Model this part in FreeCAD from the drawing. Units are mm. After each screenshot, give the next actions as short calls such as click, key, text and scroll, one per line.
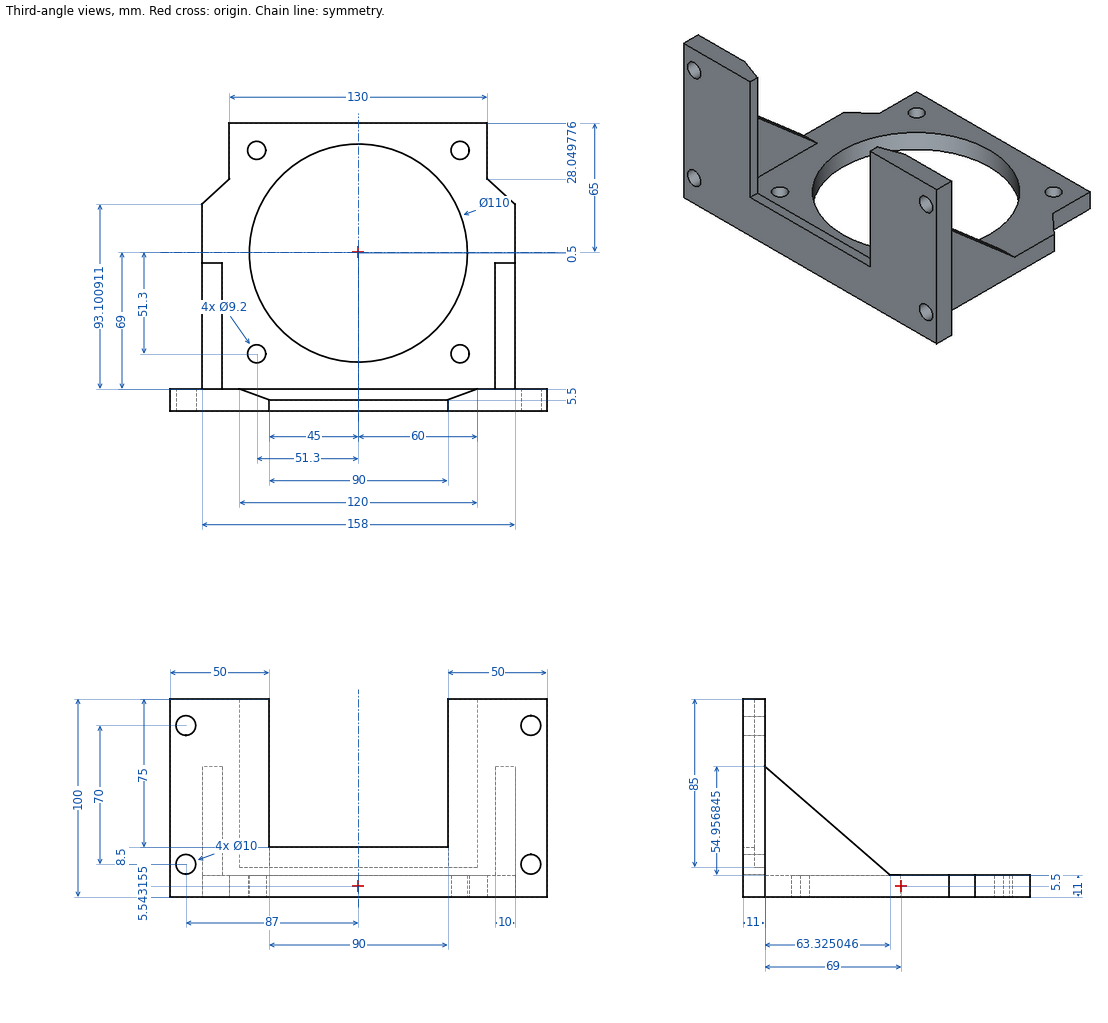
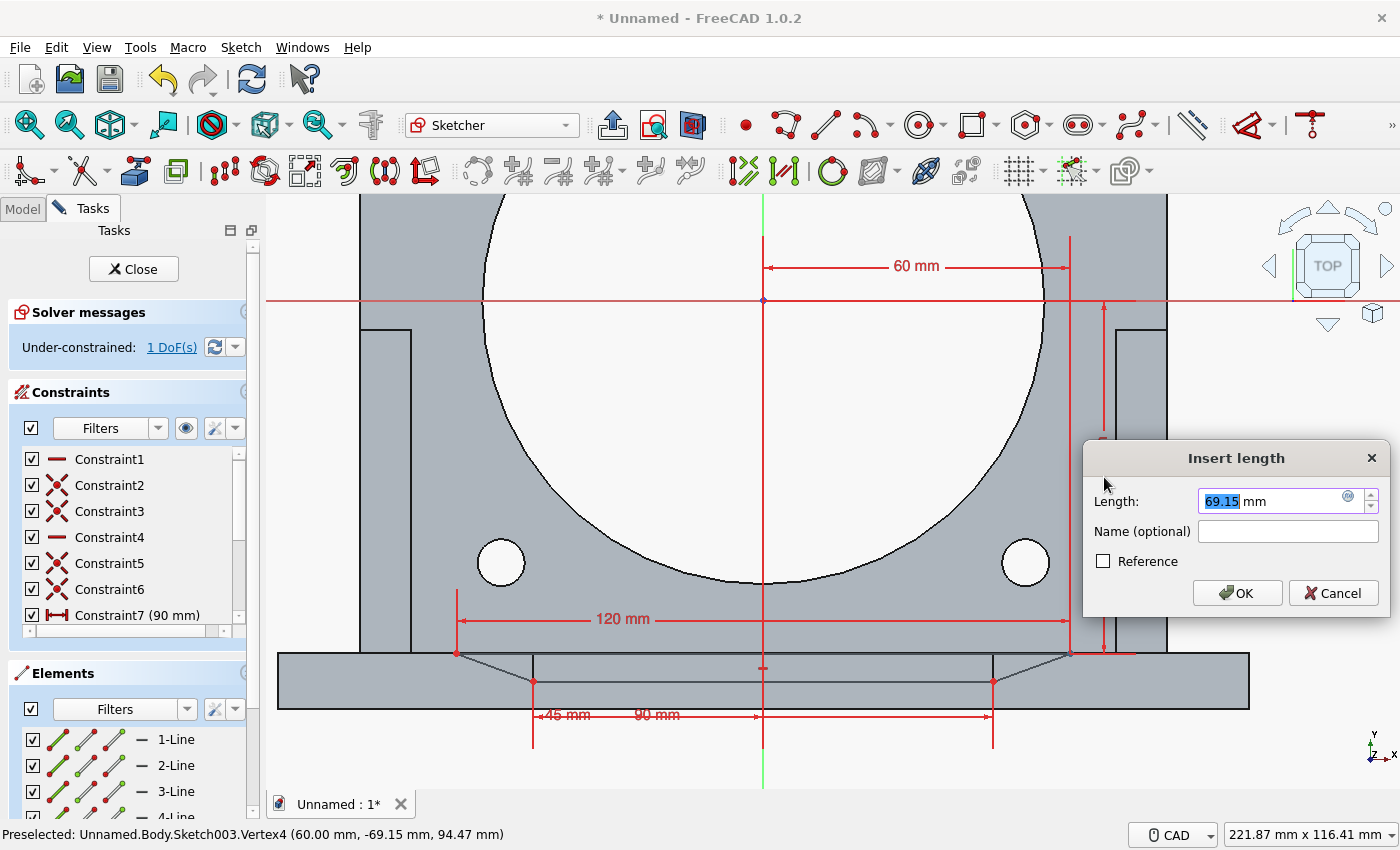
text(69)
key(Return)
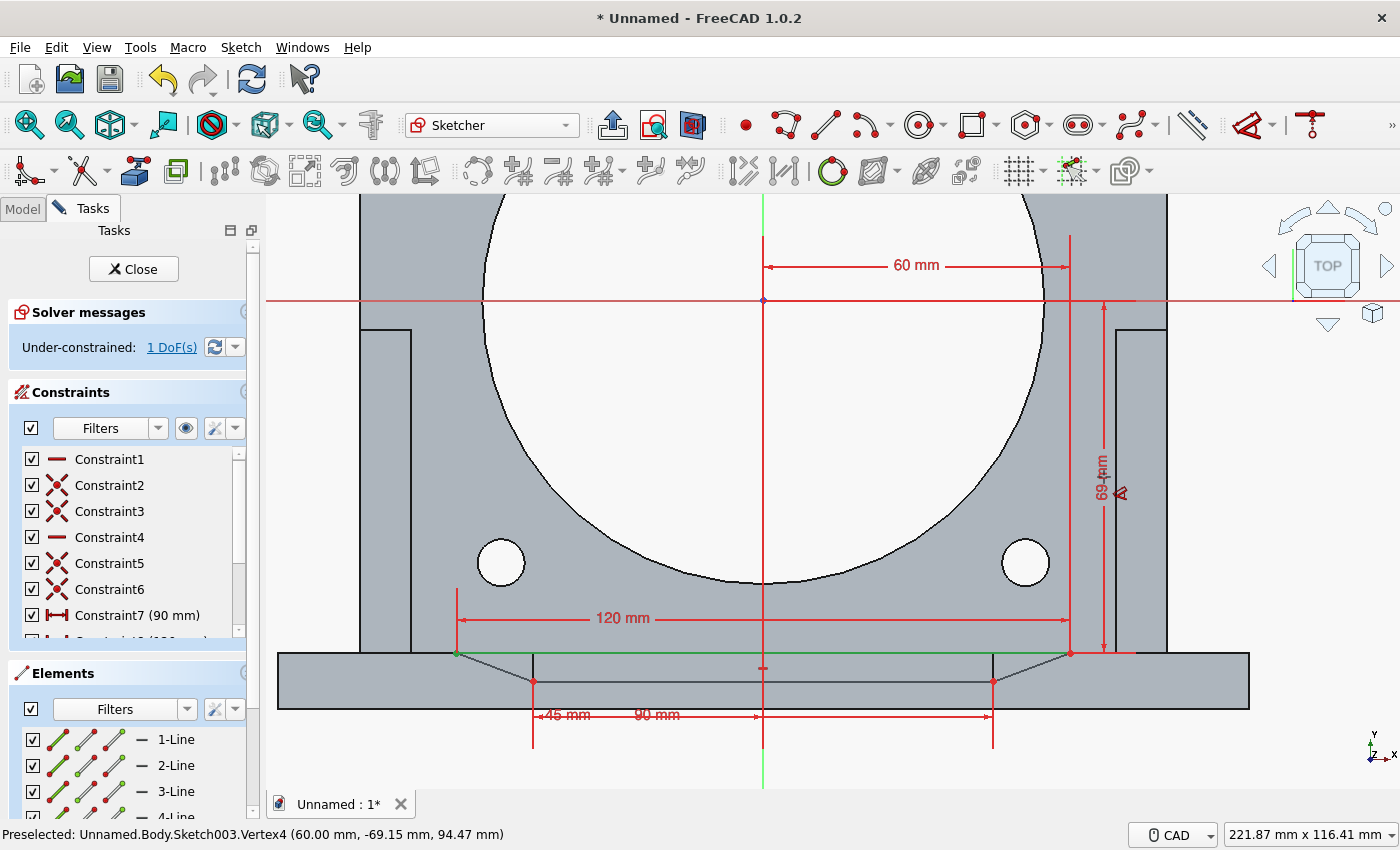
scroll(1016, 673, up, 2)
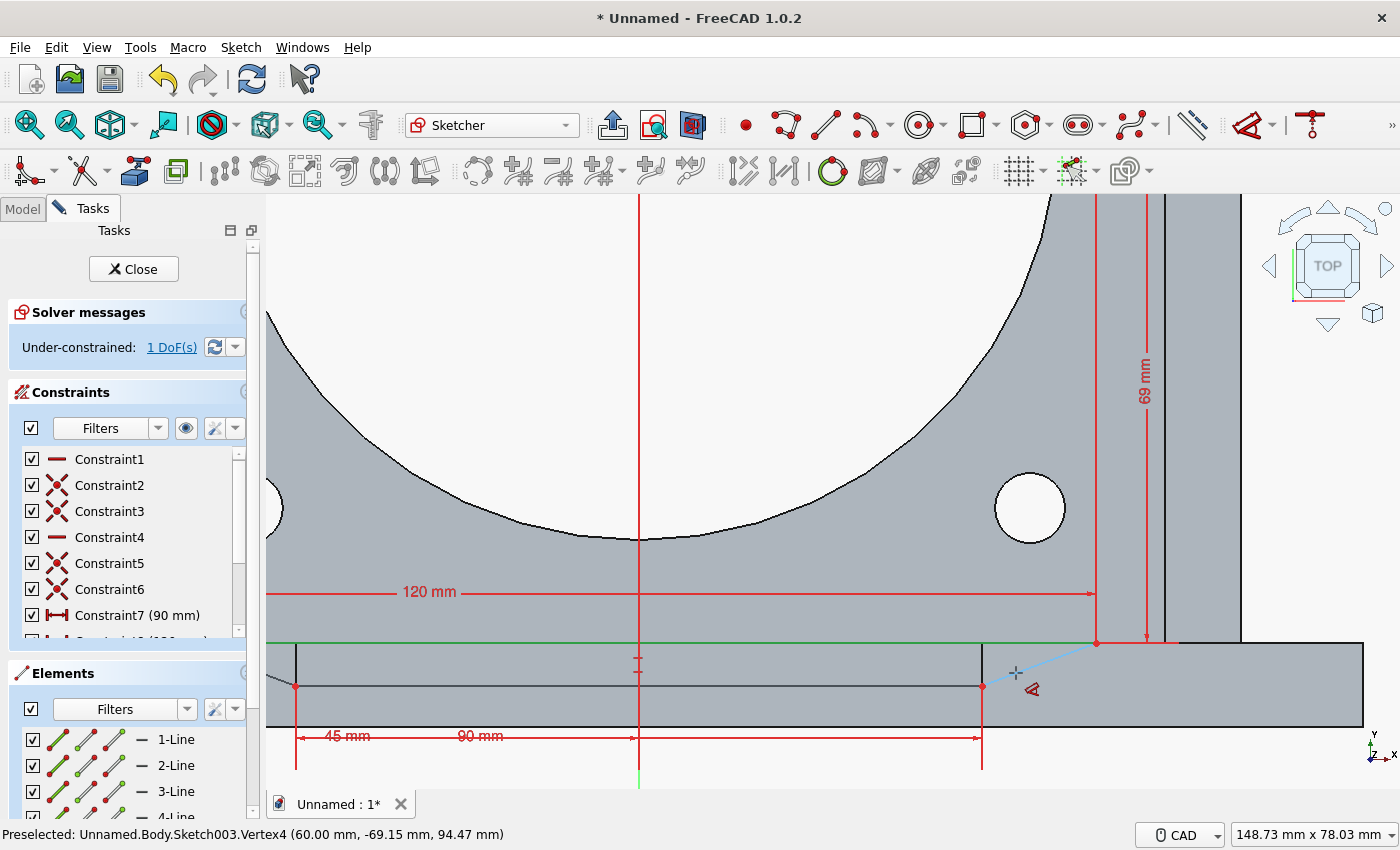
click(1016, 673)
click(1130, 665)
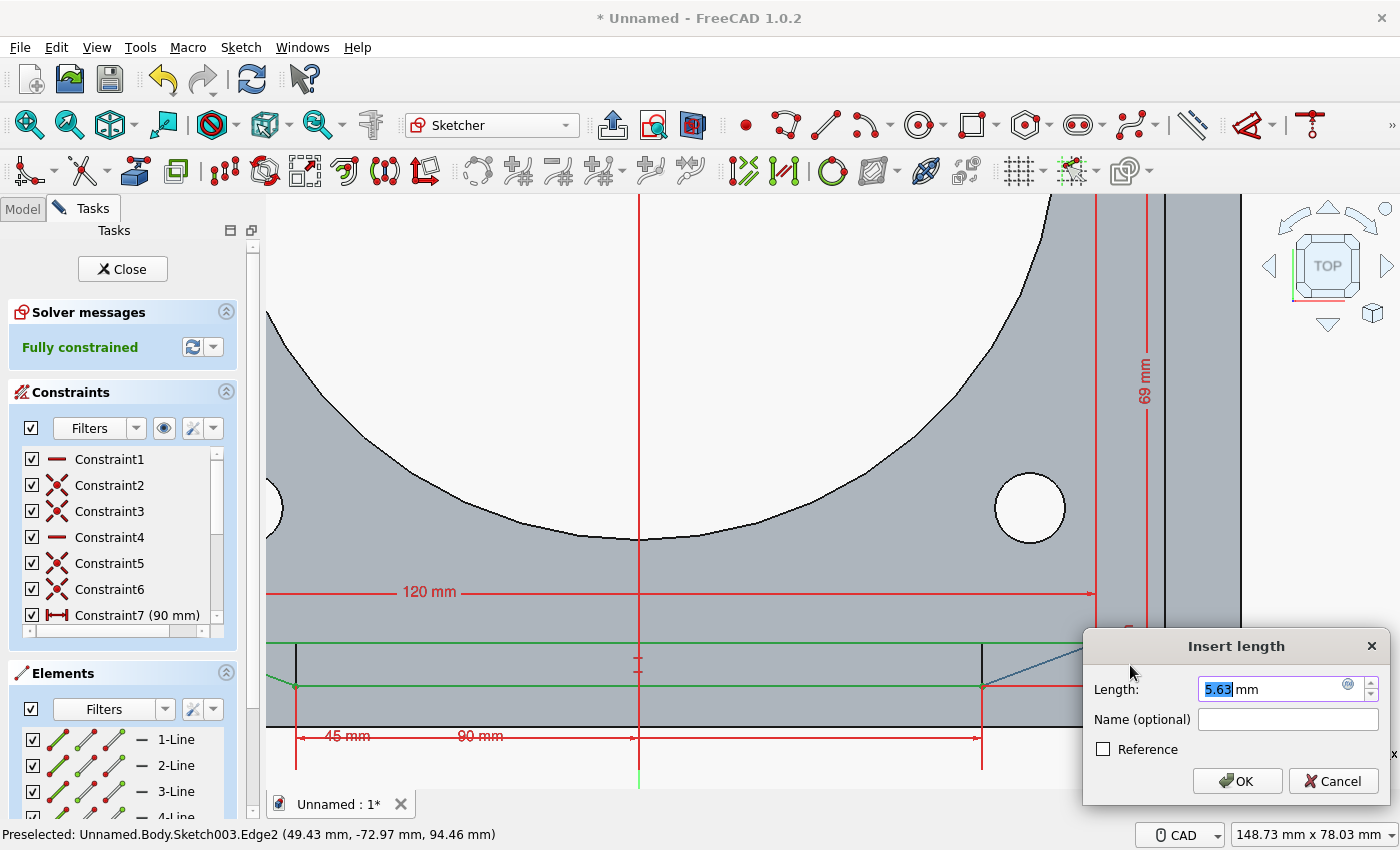
text(5.5)
key(Return)
key(Escape)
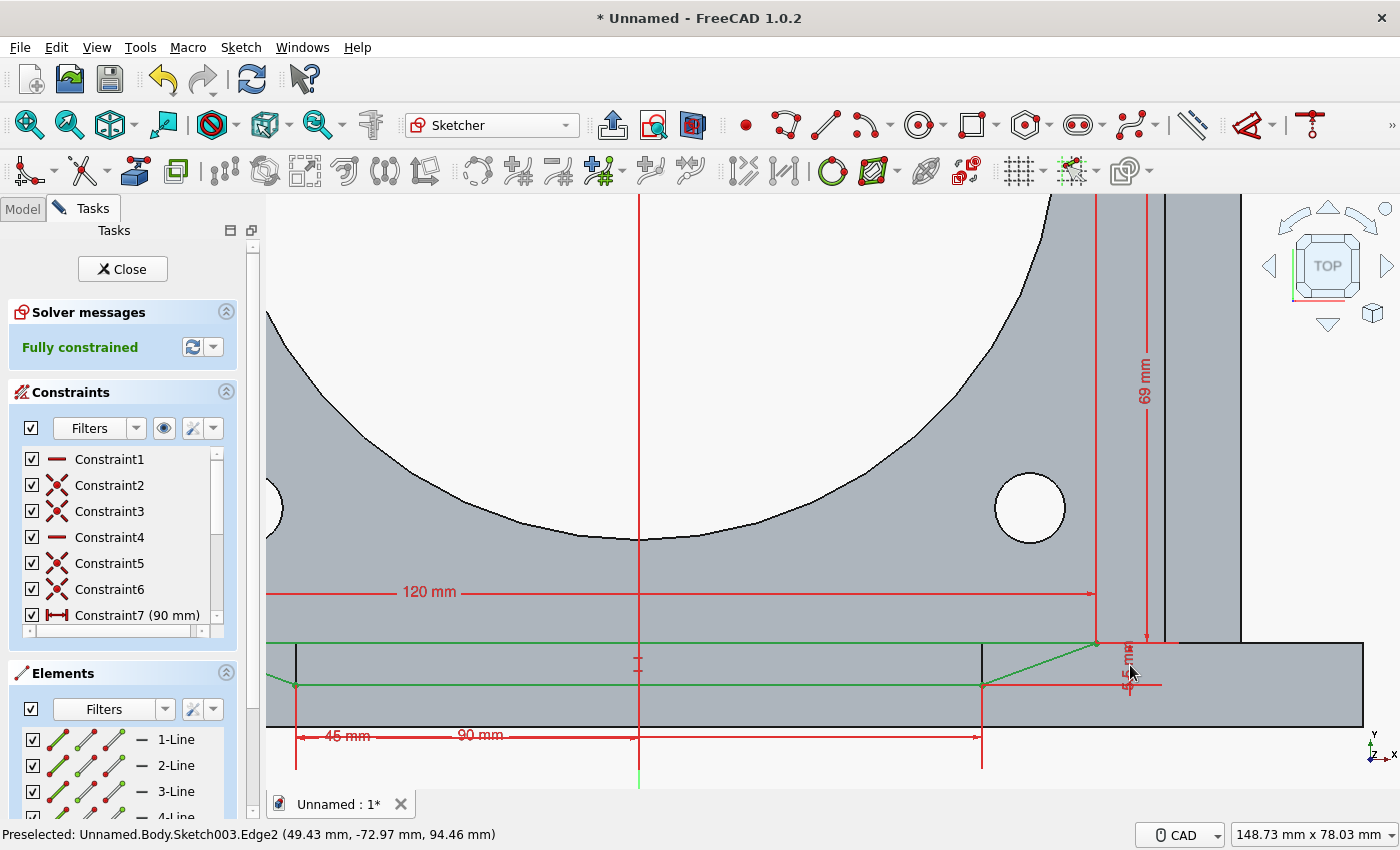
click(123, 269)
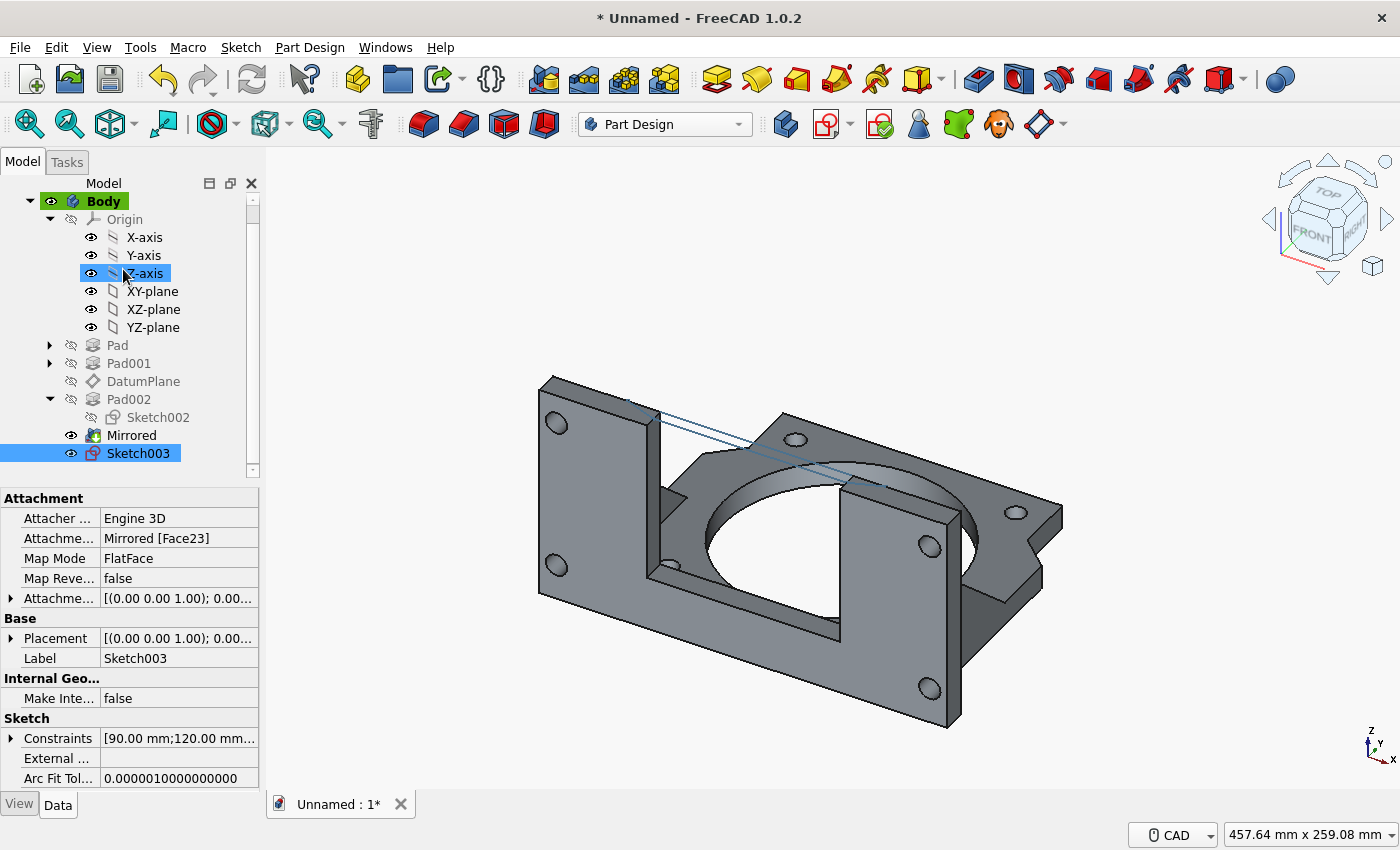
click(980, 80)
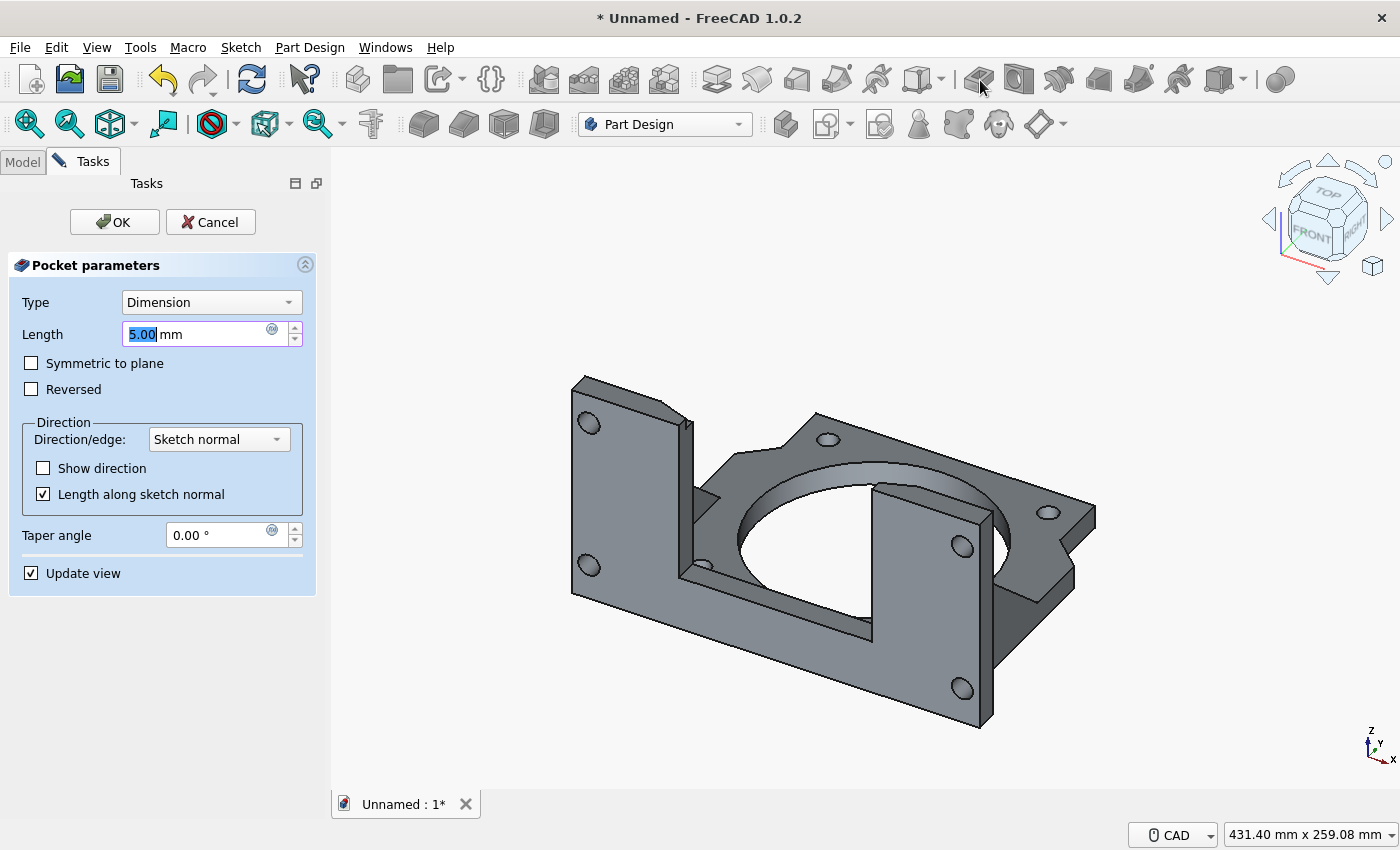
text(85)
key(Tab)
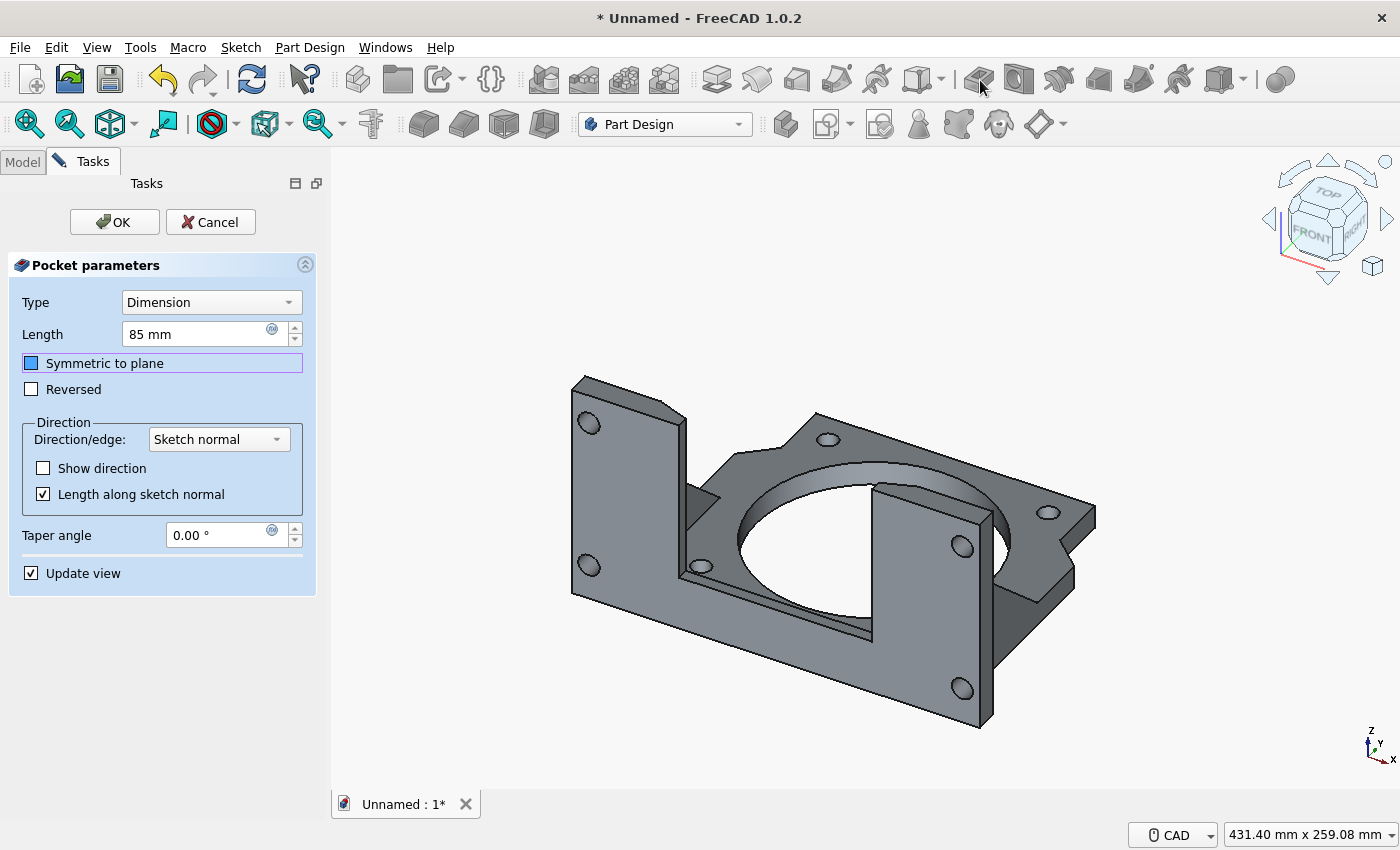
click(115, 222)